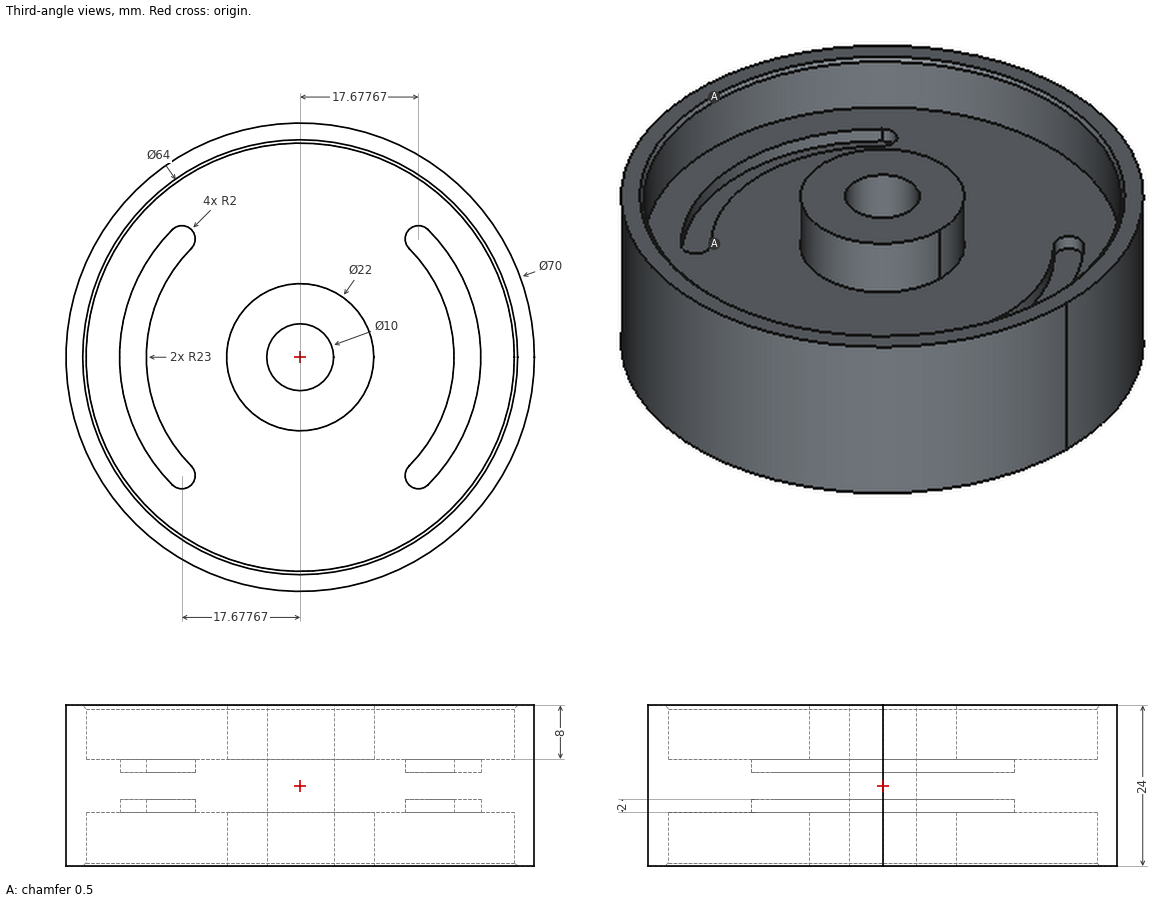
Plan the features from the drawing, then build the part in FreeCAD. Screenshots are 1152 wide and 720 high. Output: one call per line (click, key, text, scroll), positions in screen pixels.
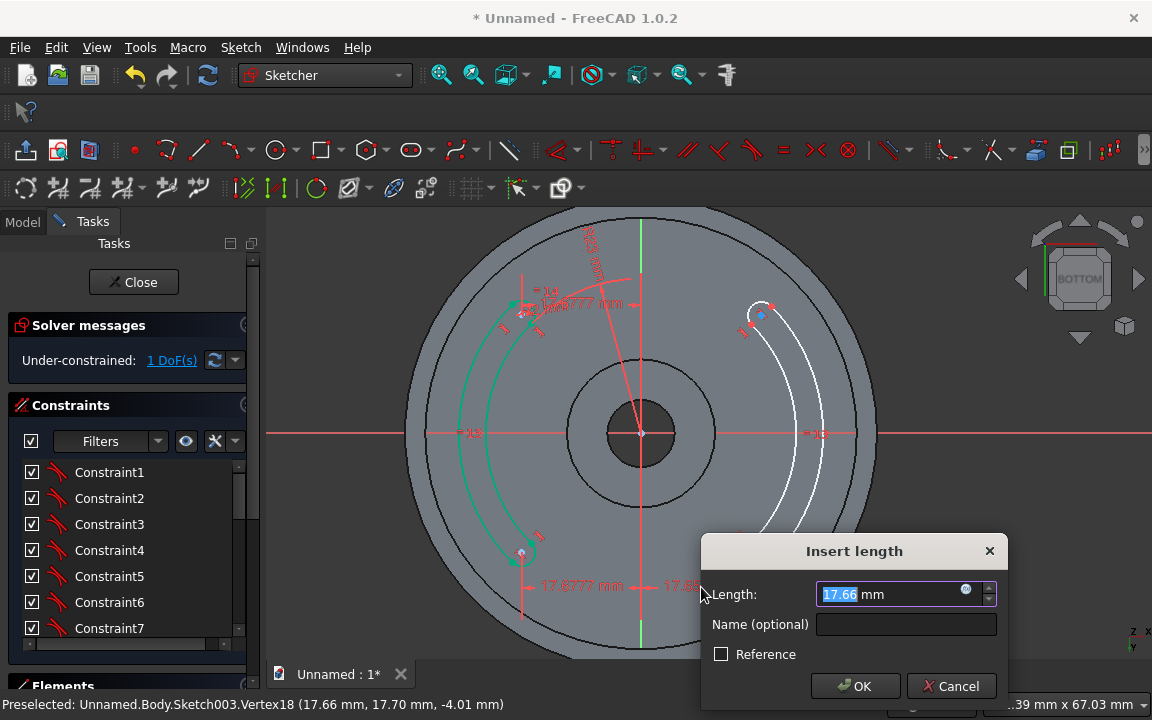
text(17.67767)
key(Return)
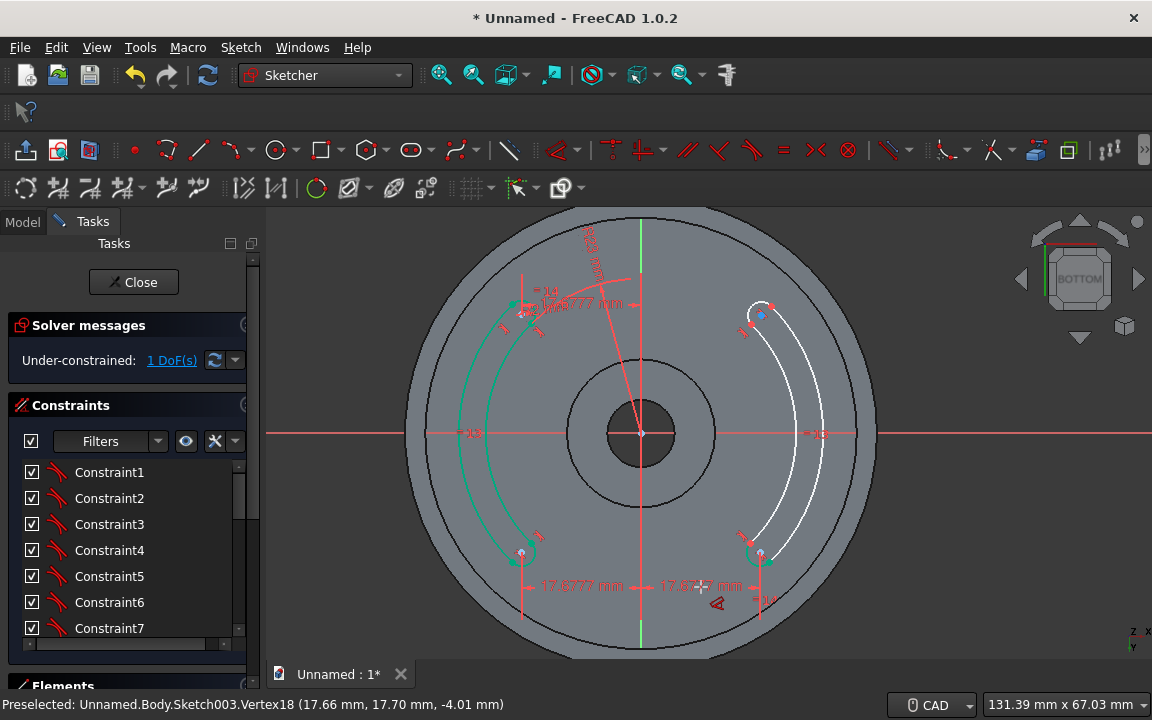
click(761, 315)
click(701, 281)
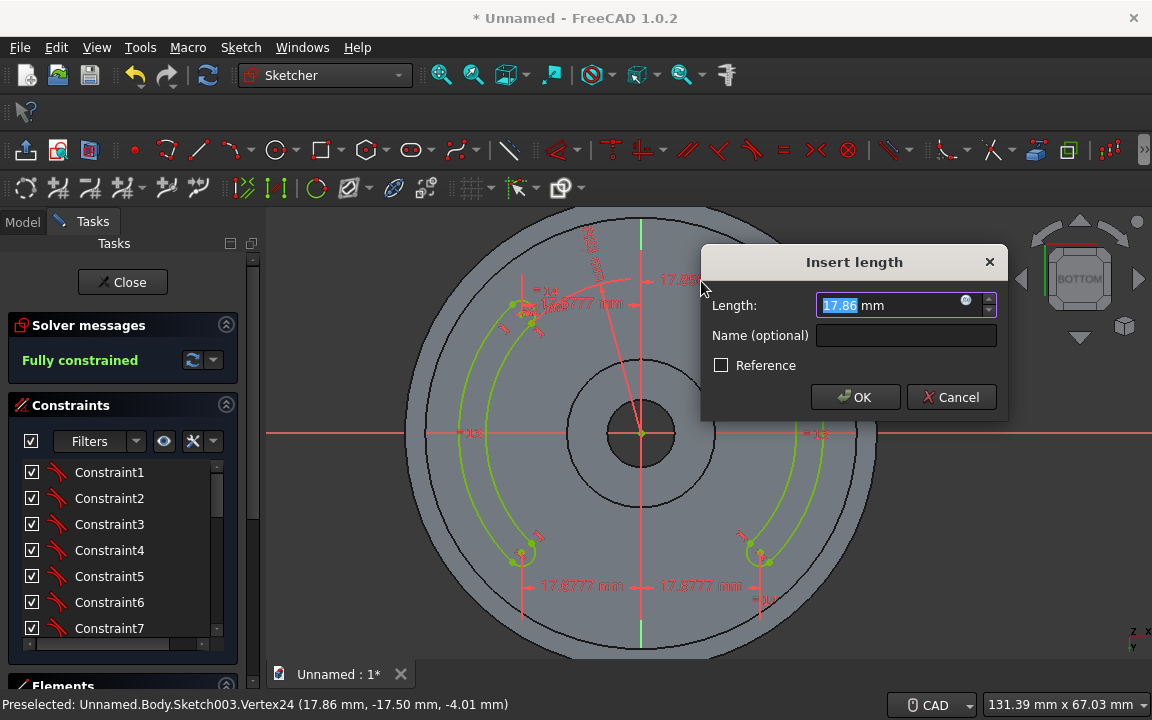
text(17.67767)
key(Return)
key(Escape)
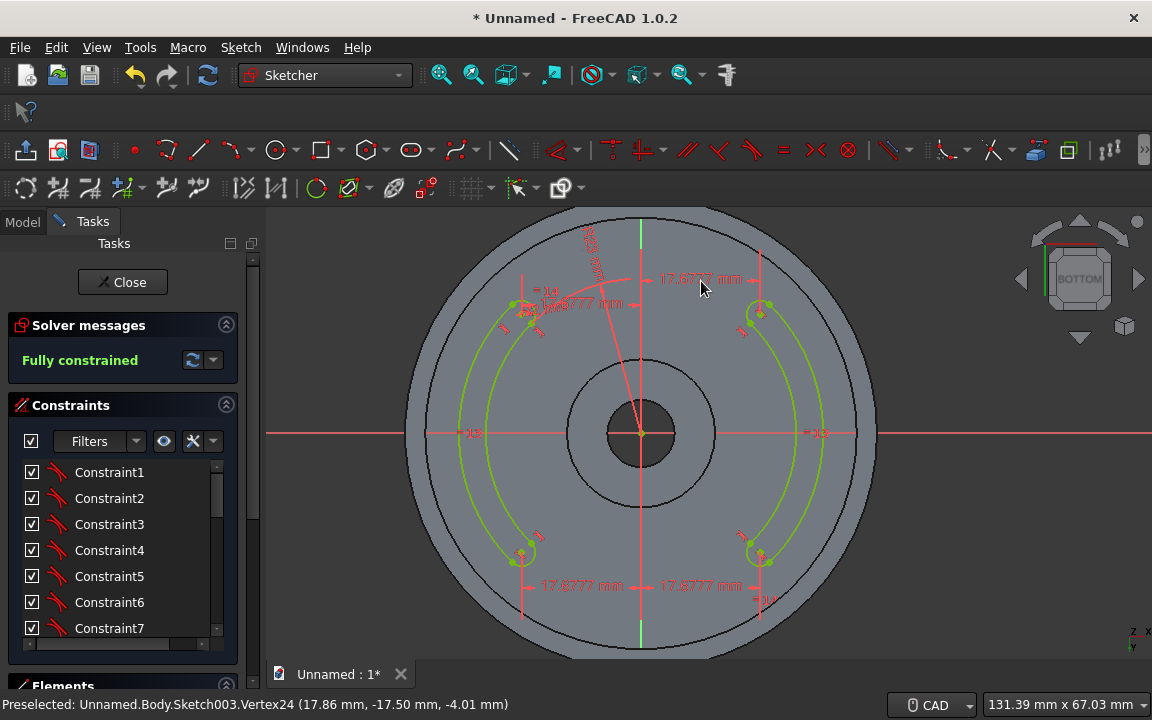
click(123, 282)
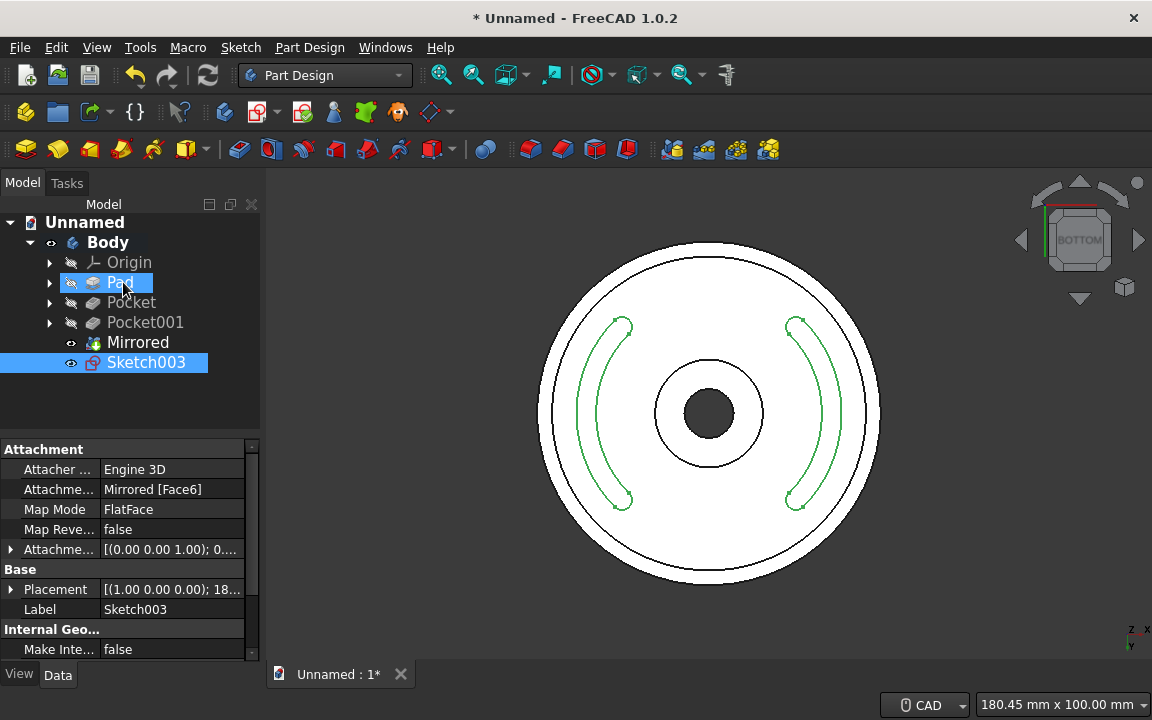
click(240, 150)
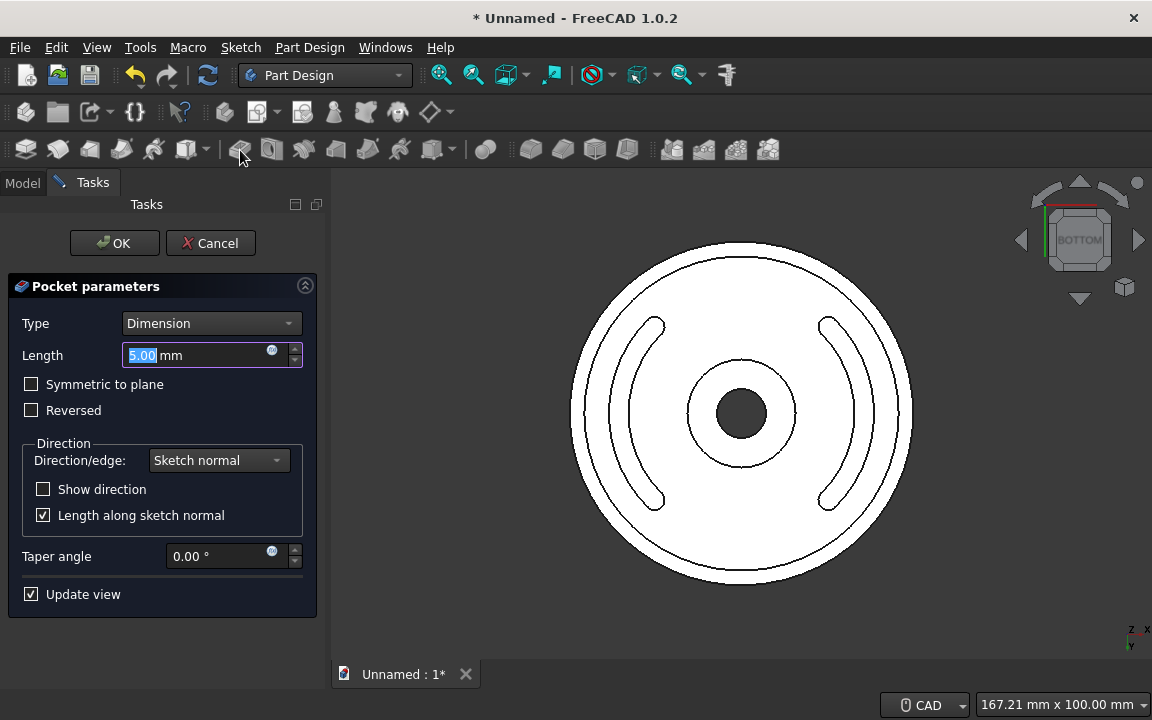
text(2)
key(Tab)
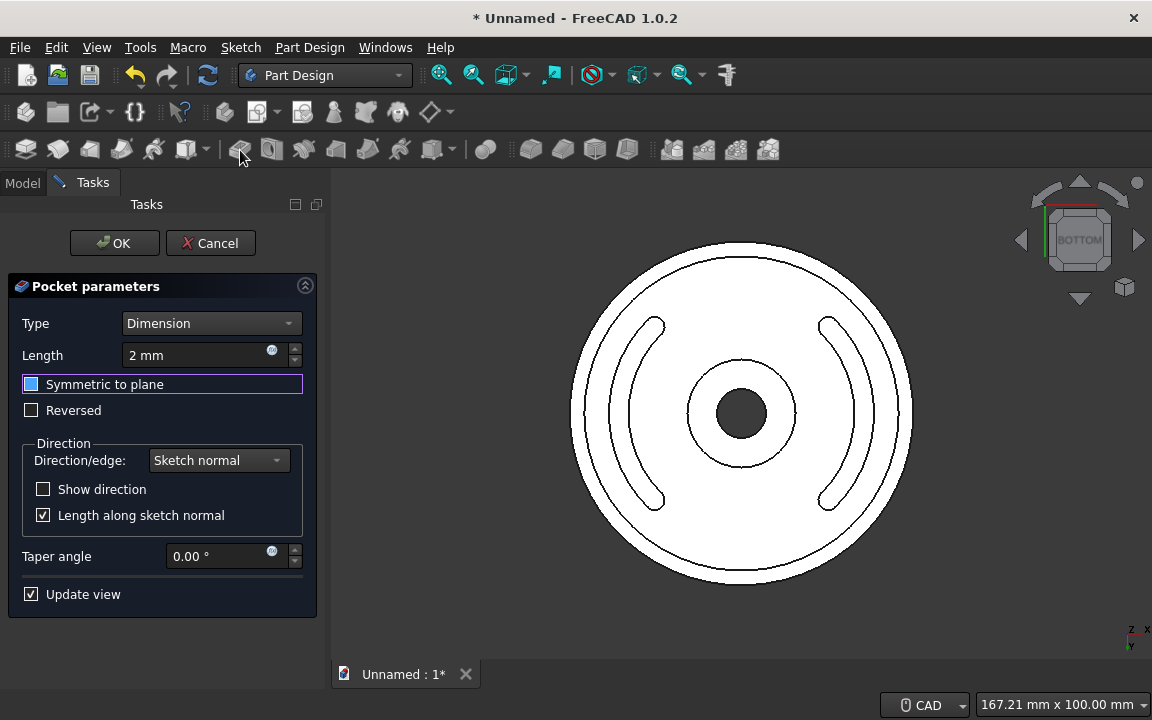
click(115, 243)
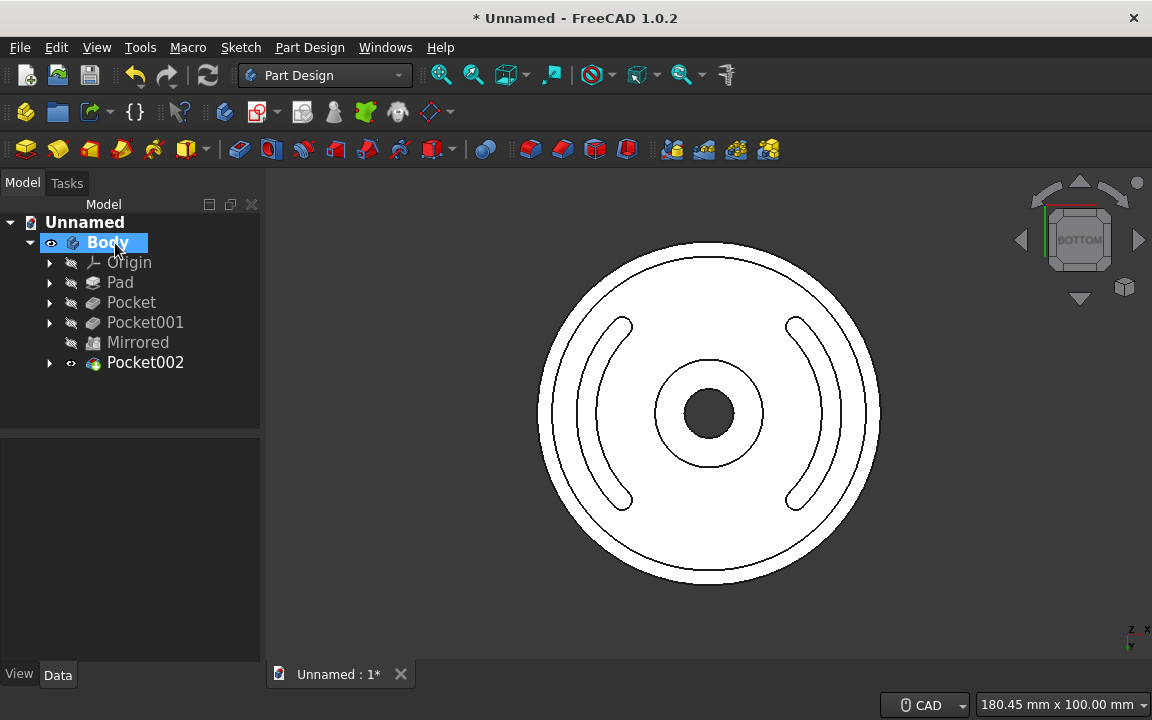
click(116, 363)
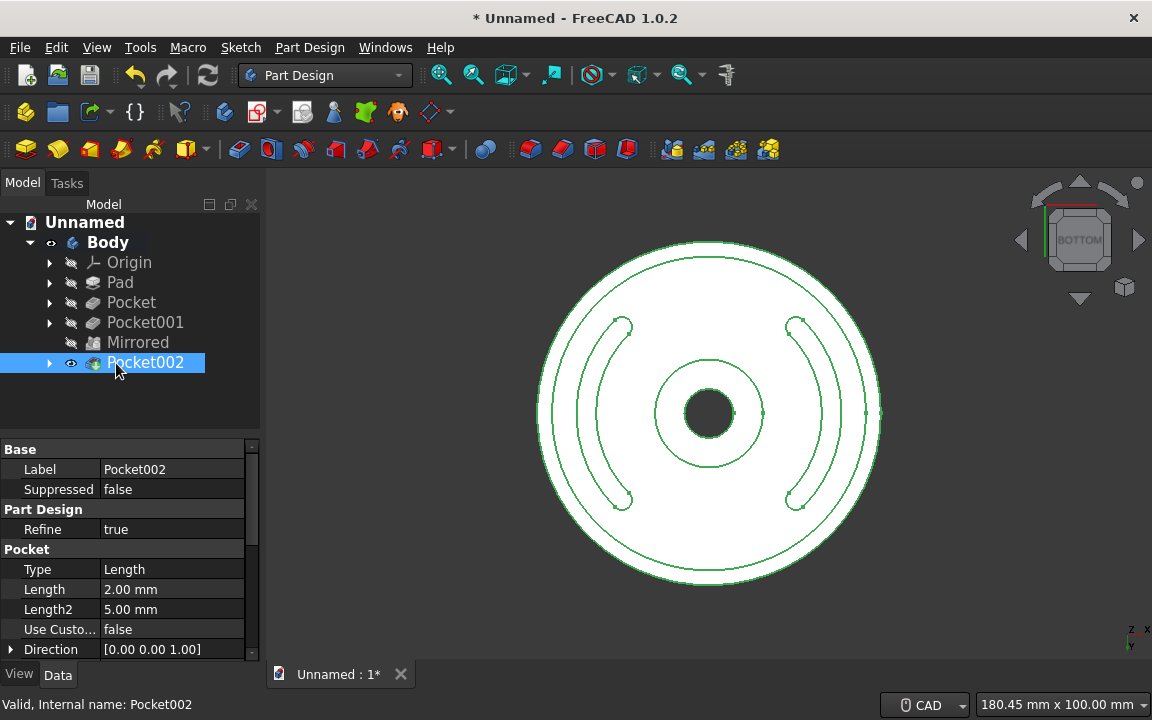
click(672, 150)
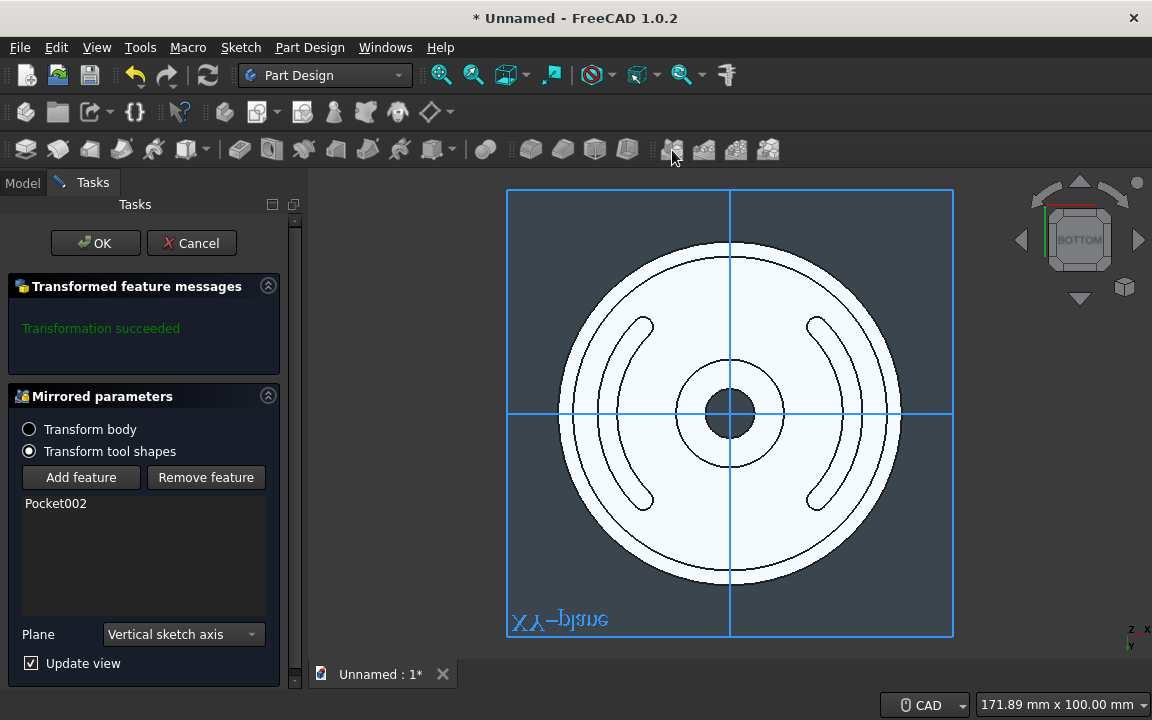
click(184, 634)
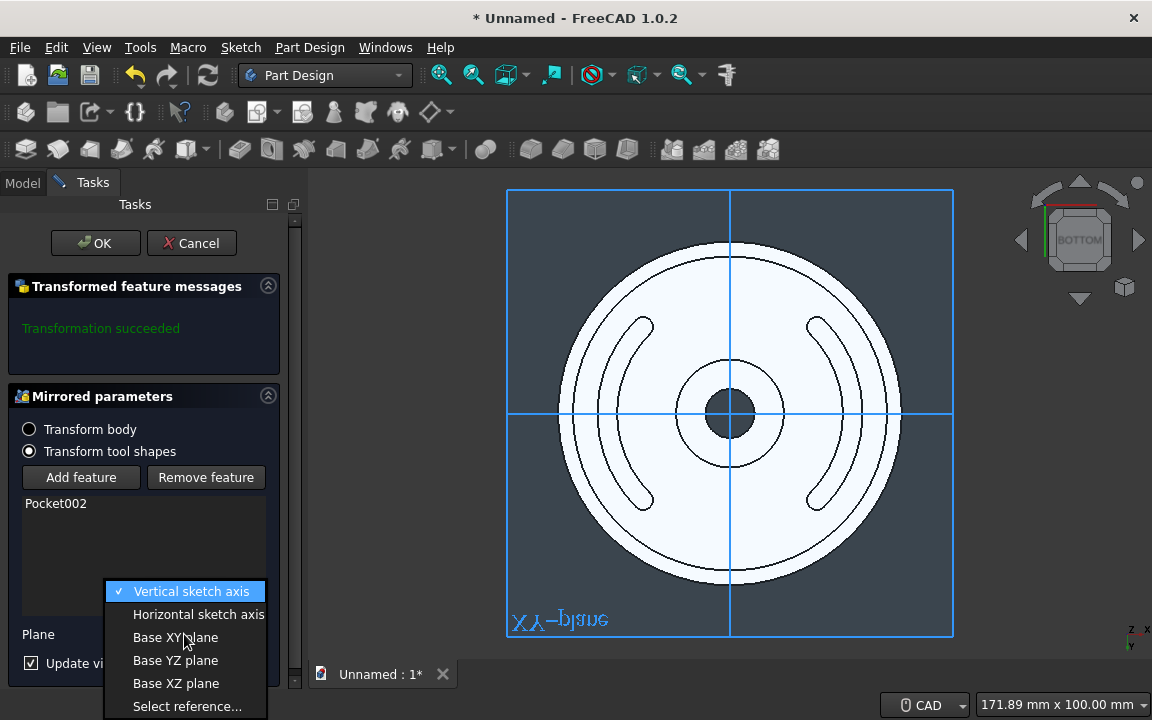
click(184, 638)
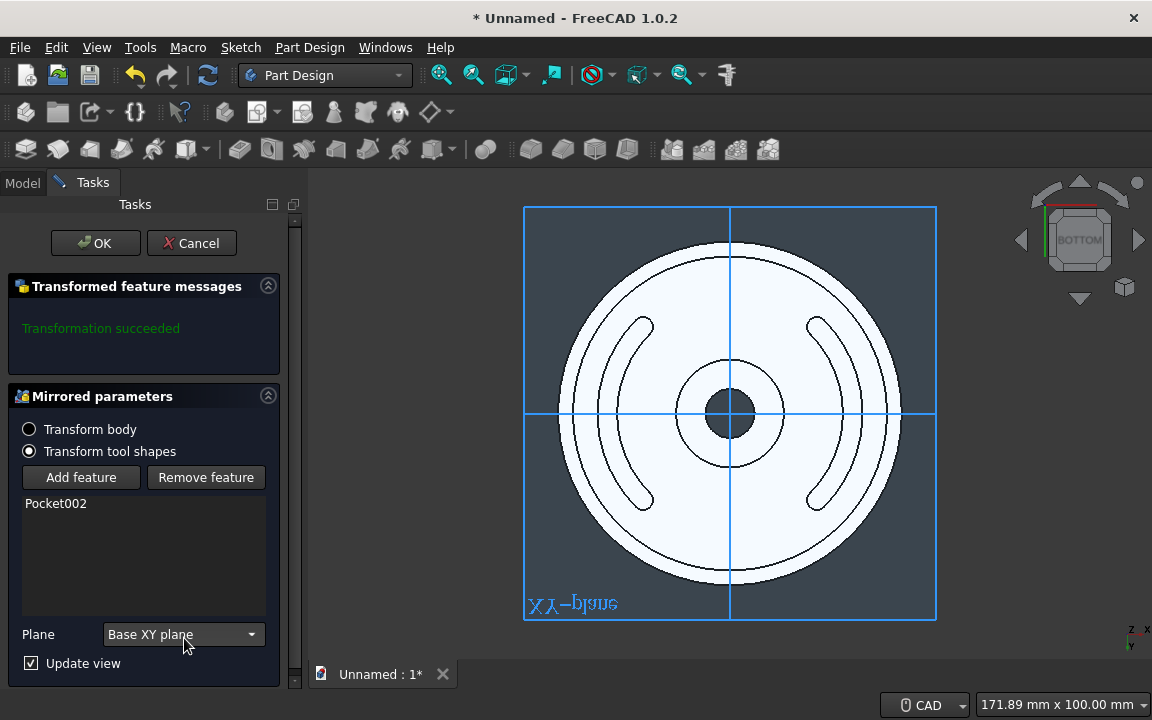
click(96, 243)